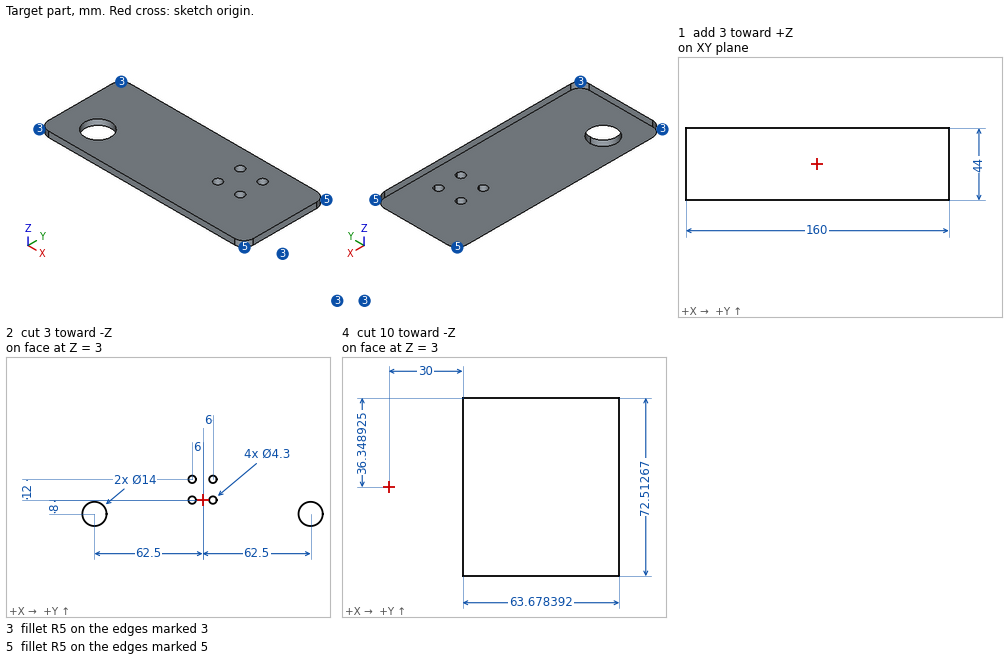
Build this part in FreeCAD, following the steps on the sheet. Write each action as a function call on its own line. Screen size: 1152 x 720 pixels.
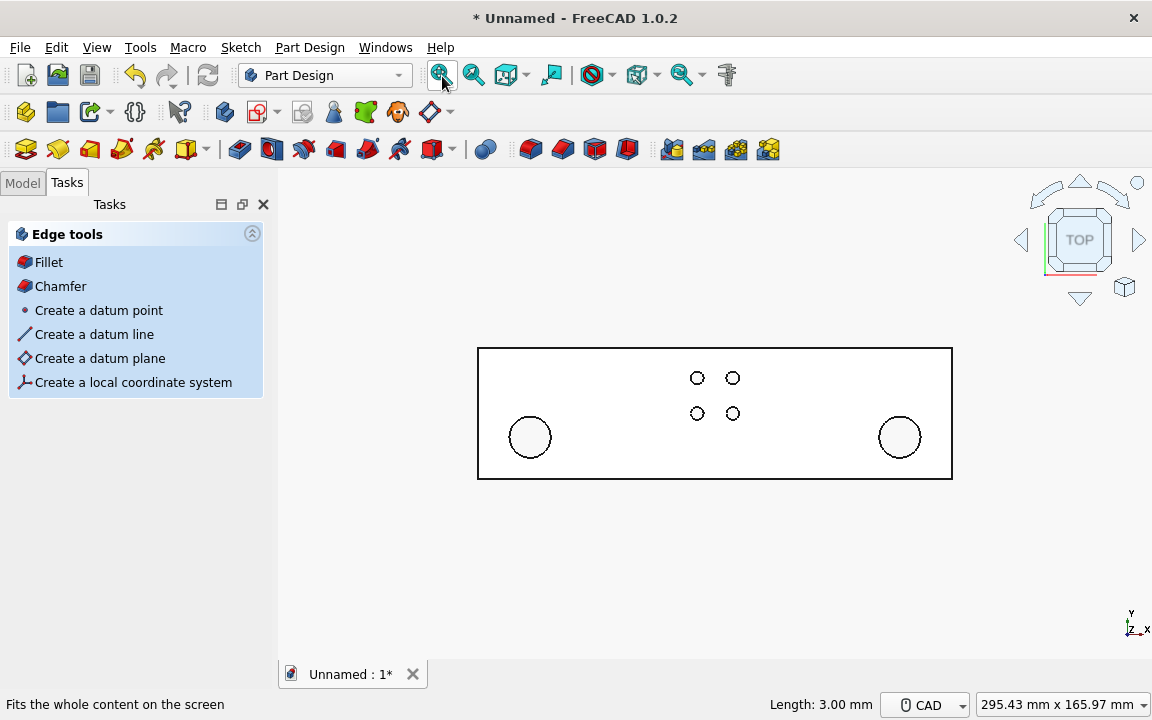
key(1)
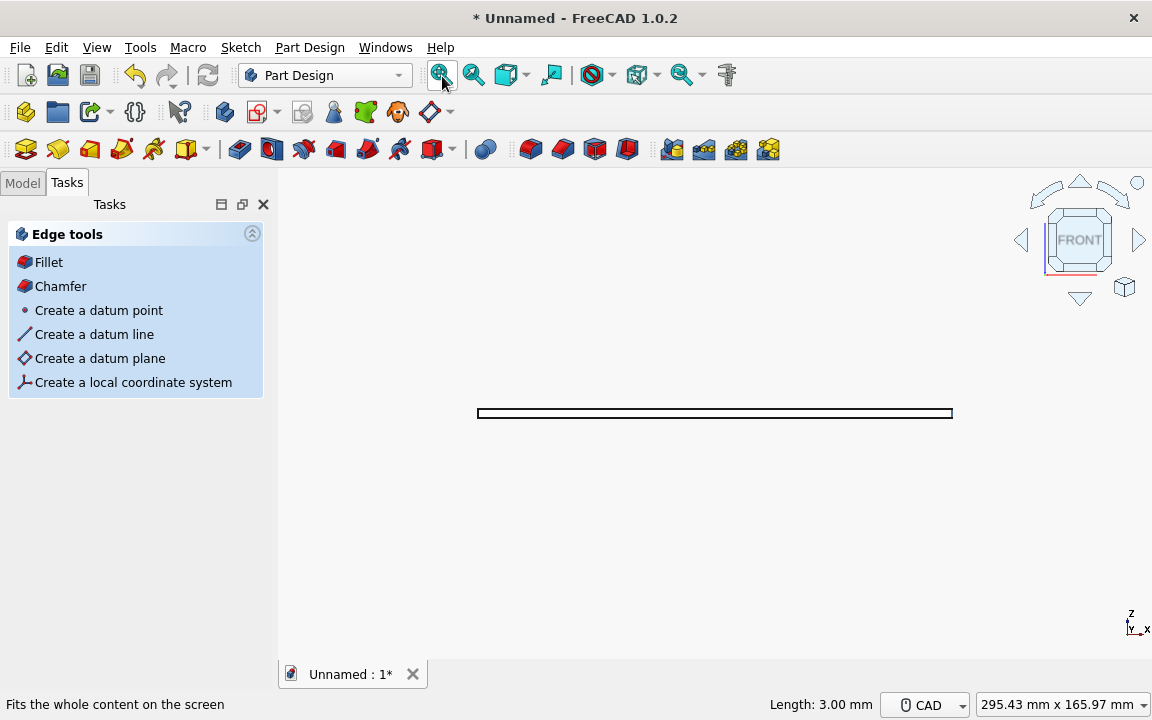
scroll(478, 413, up, 8)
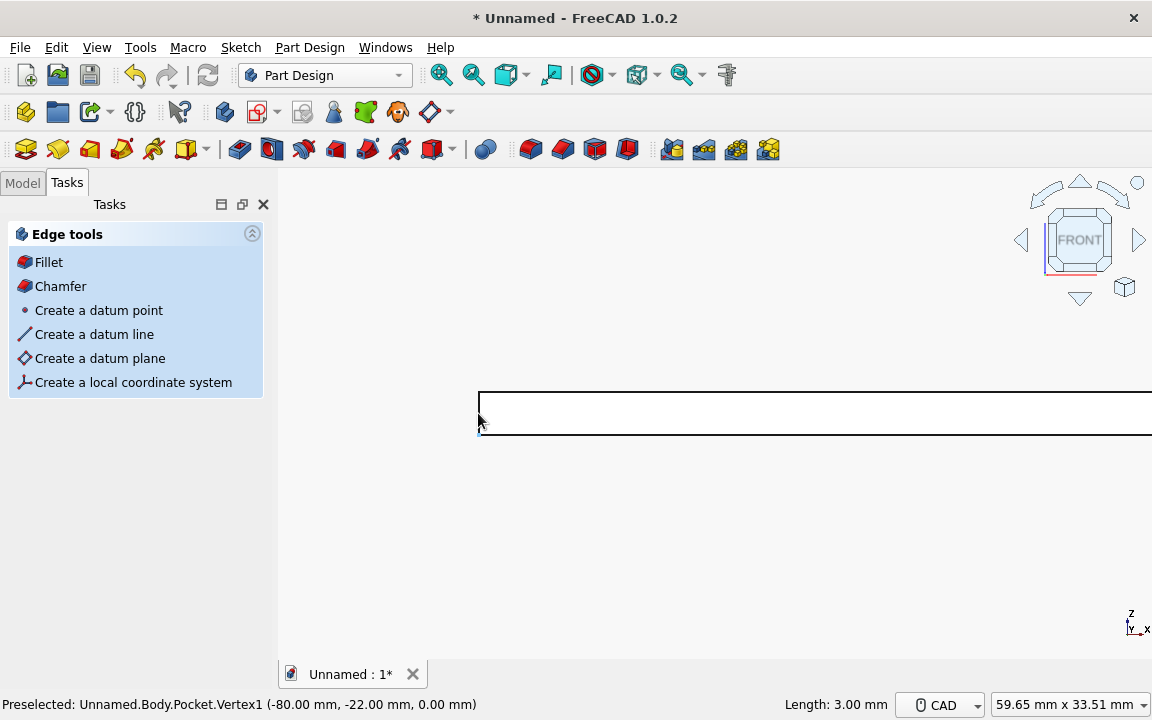
click(479, 413, ctrl)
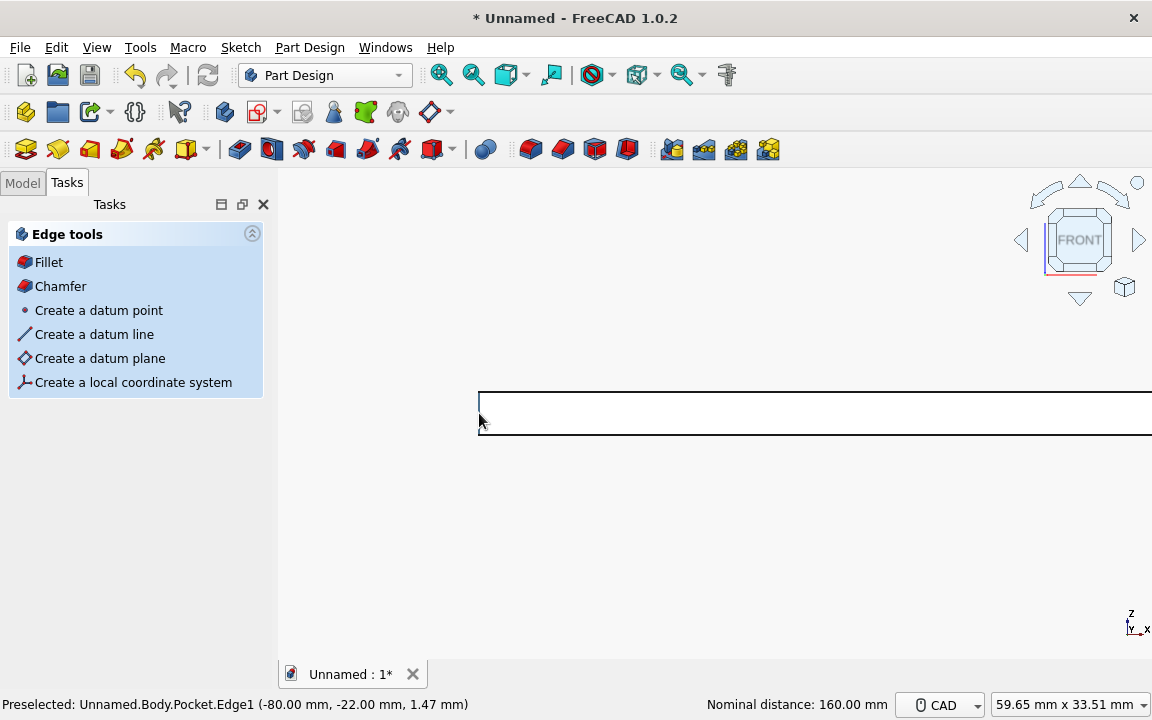
click(442, 76)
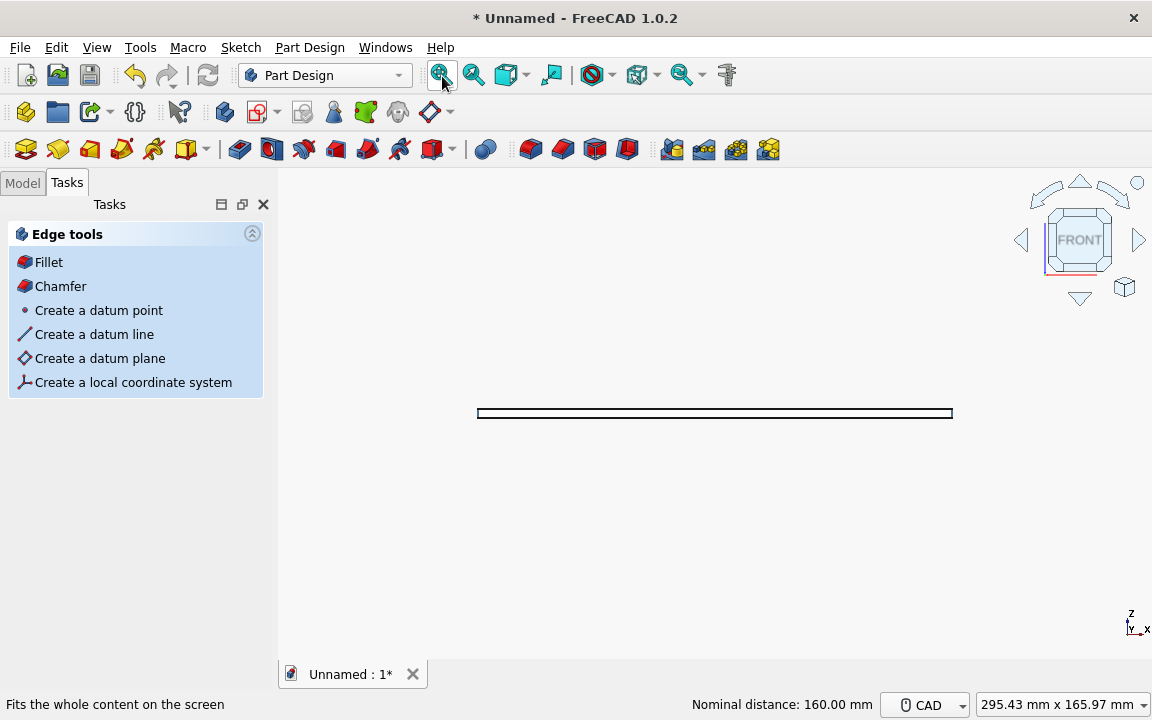
key(3)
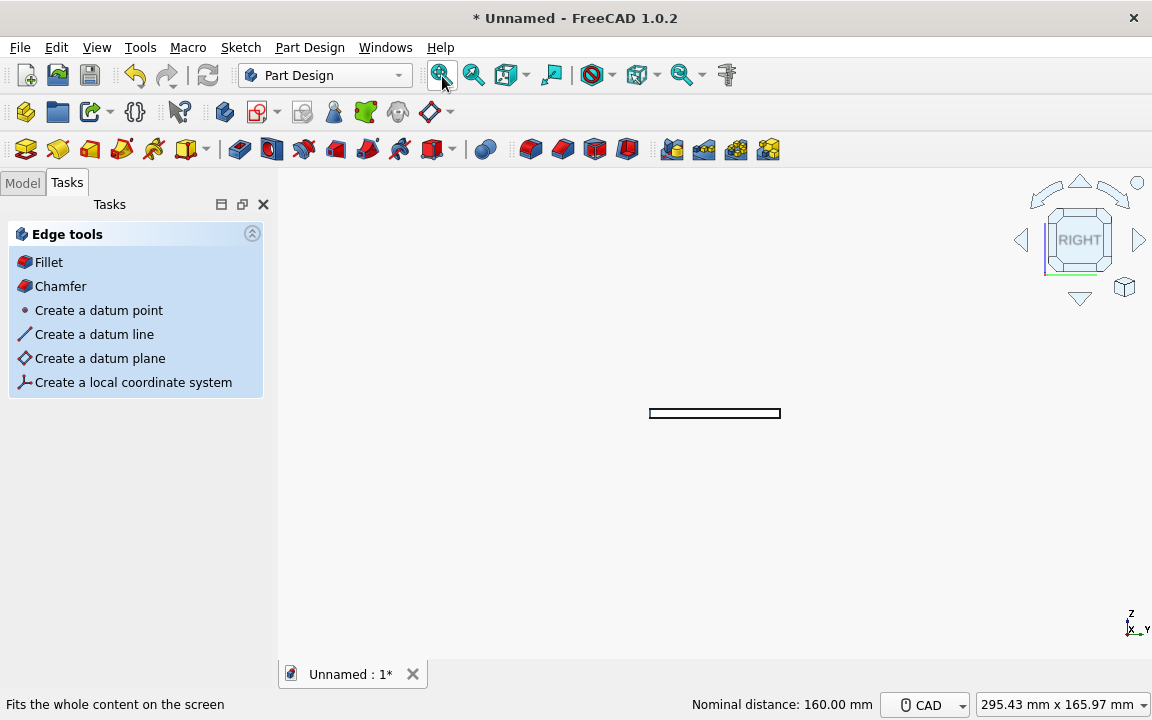
key(v)
key(f)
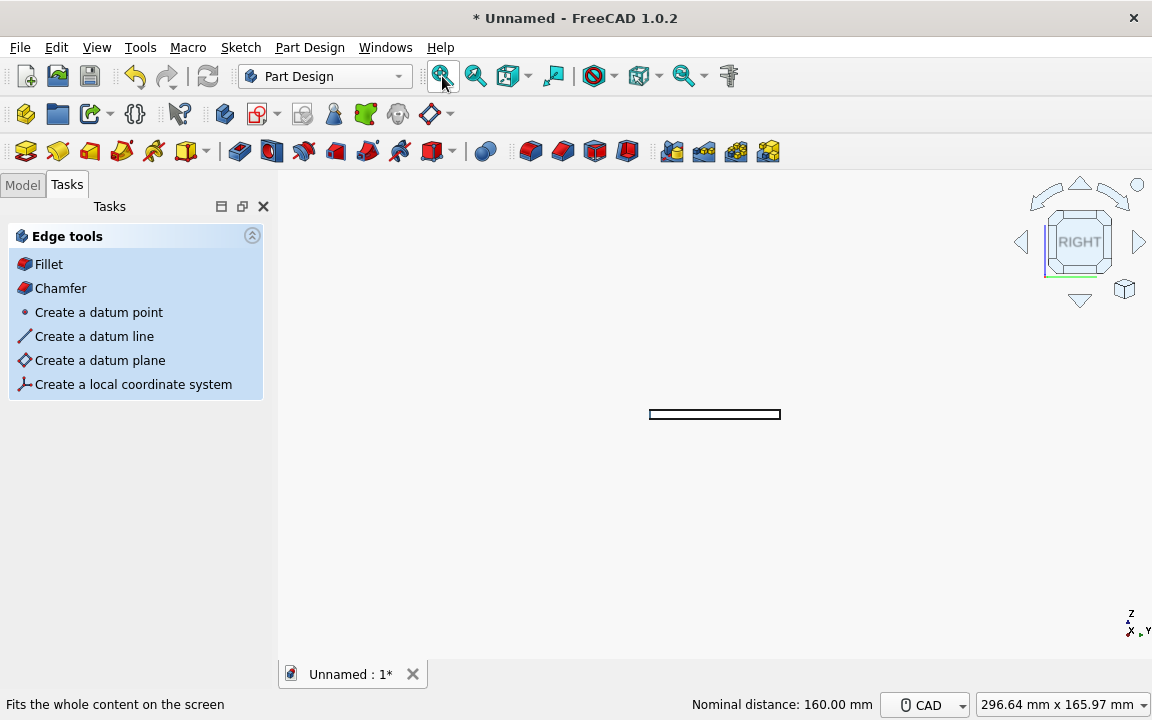
scroll(780, 413, up, 8)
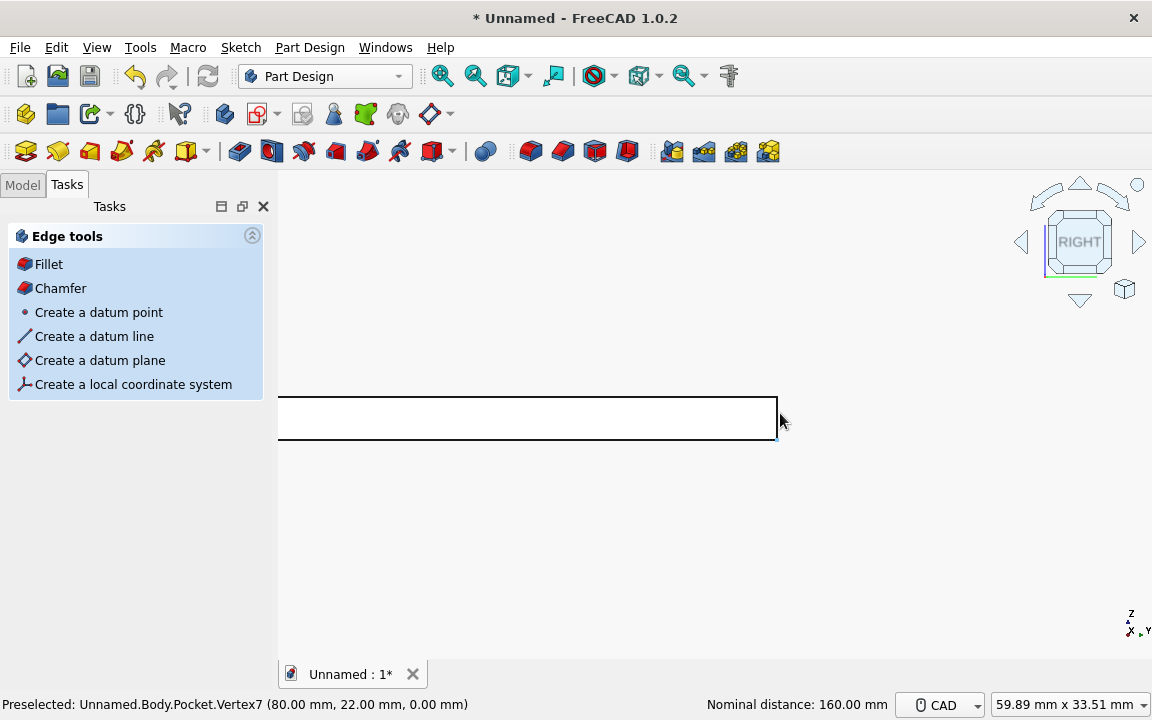
click(777, 417, ctrl)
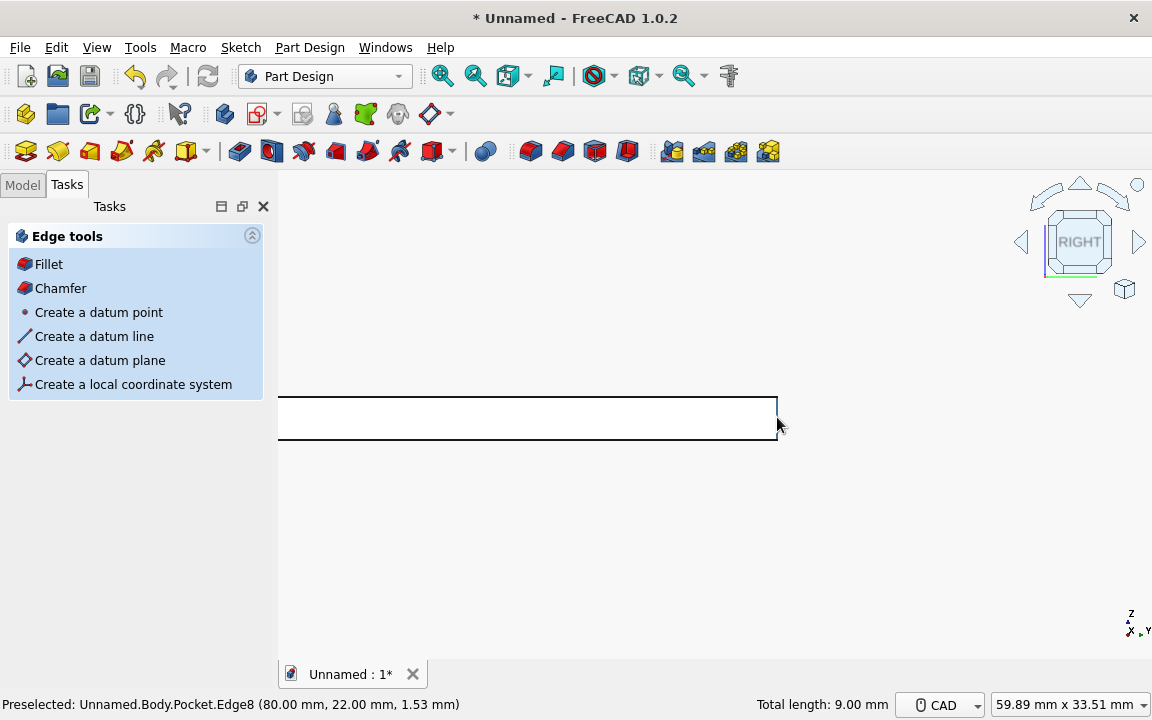
click(444, 76)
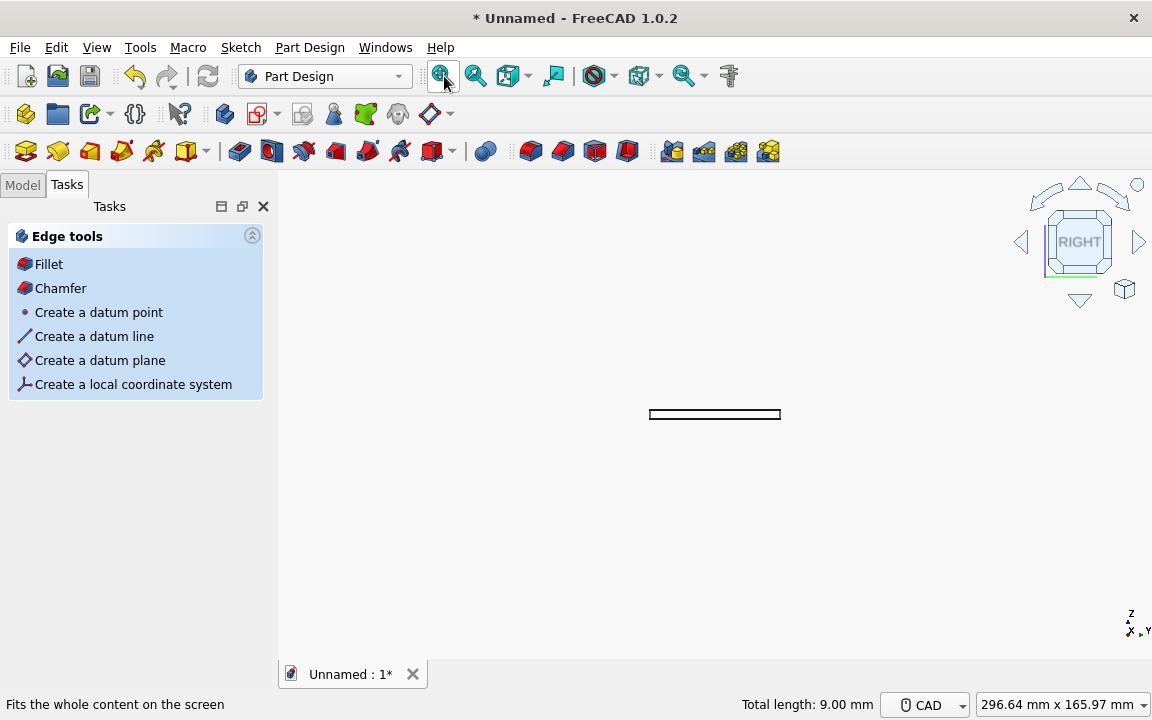
key(5)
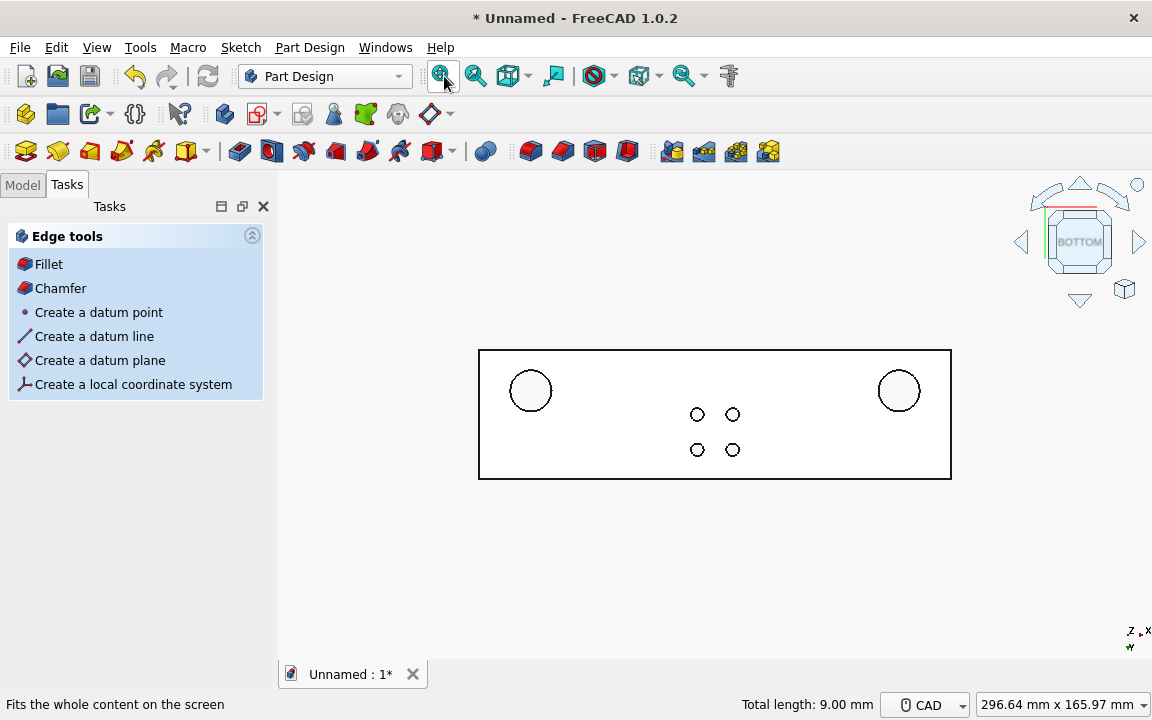
scroll(479, 478, up, 8)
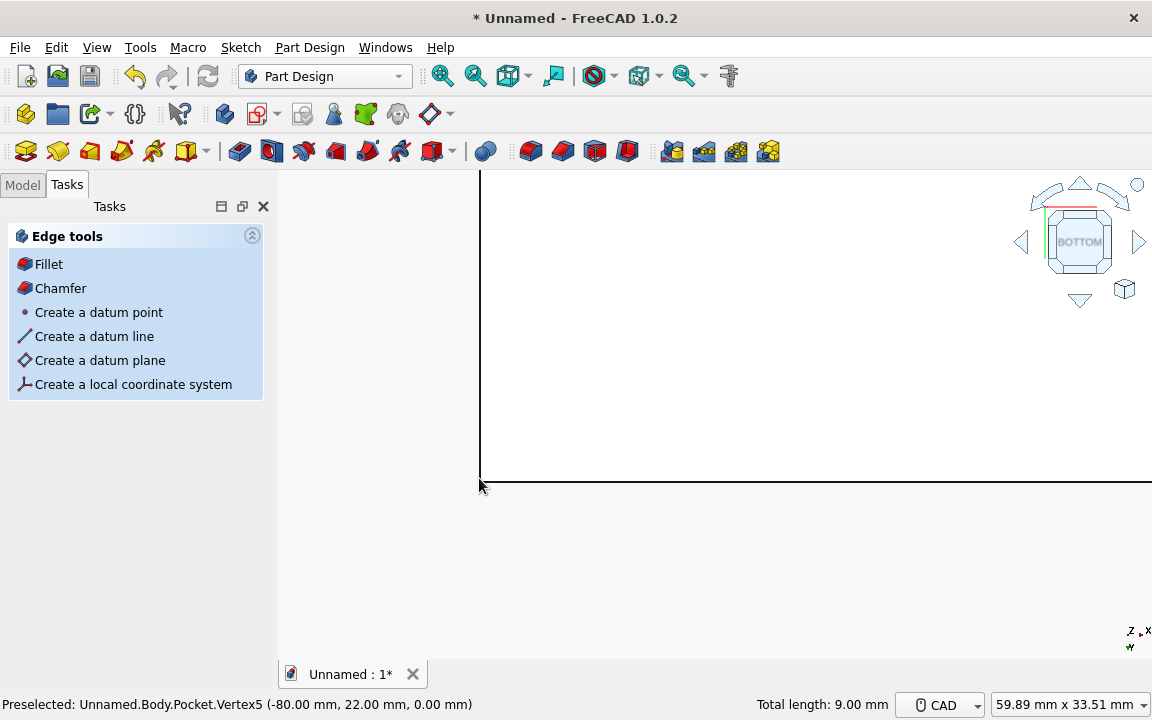
key(v)
key(f)